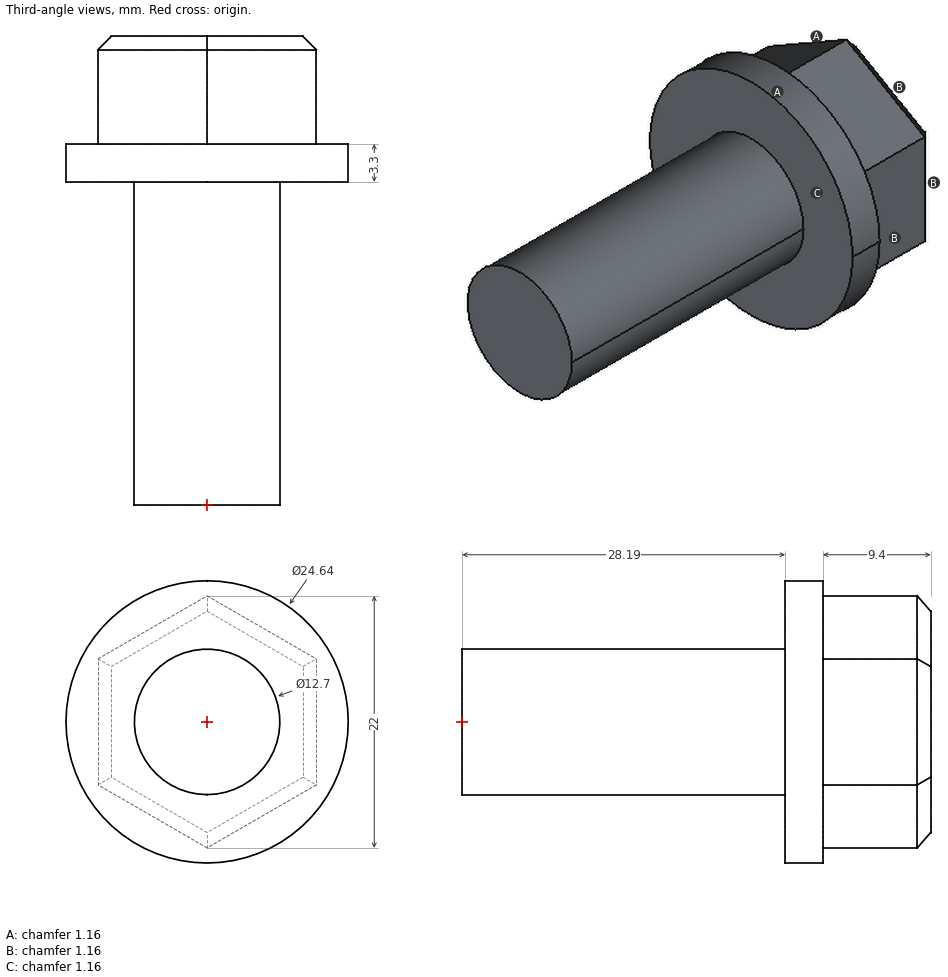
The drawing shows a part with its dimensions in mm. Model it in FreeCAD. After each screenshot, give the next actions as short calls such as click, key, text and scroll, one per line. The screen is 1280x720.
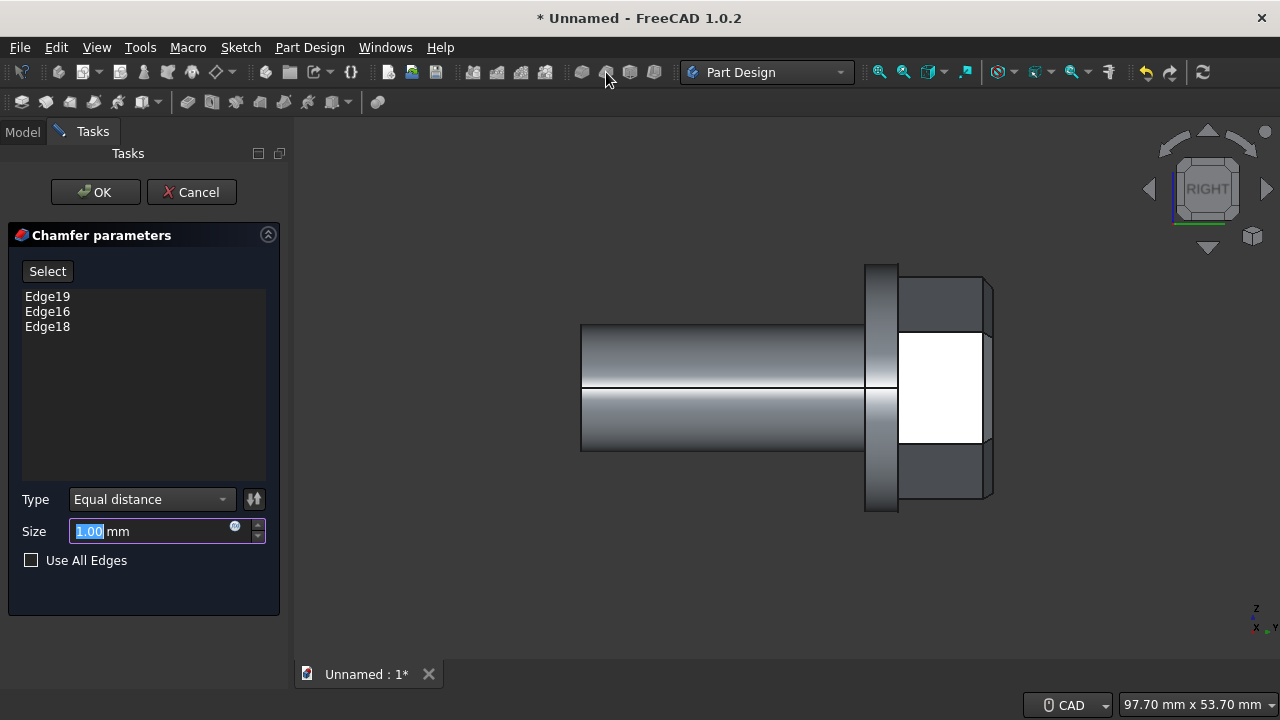
text(1.16)
key(Tab)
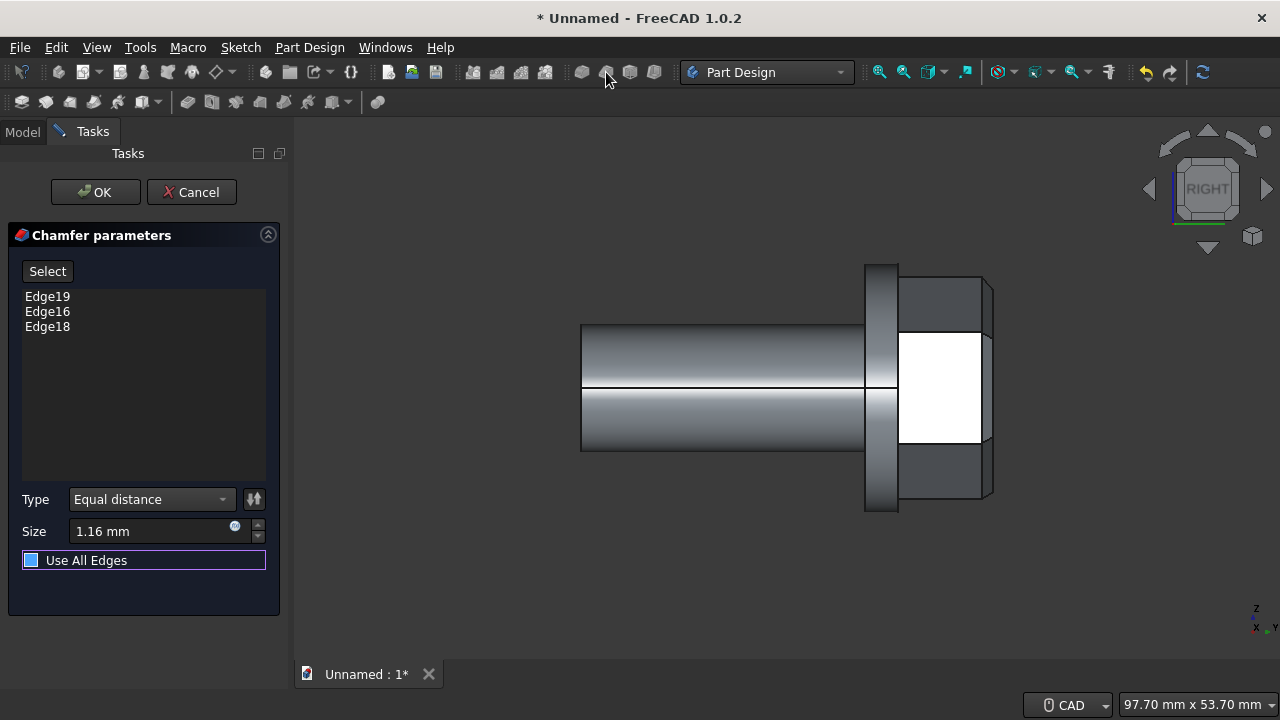
click(96, 192)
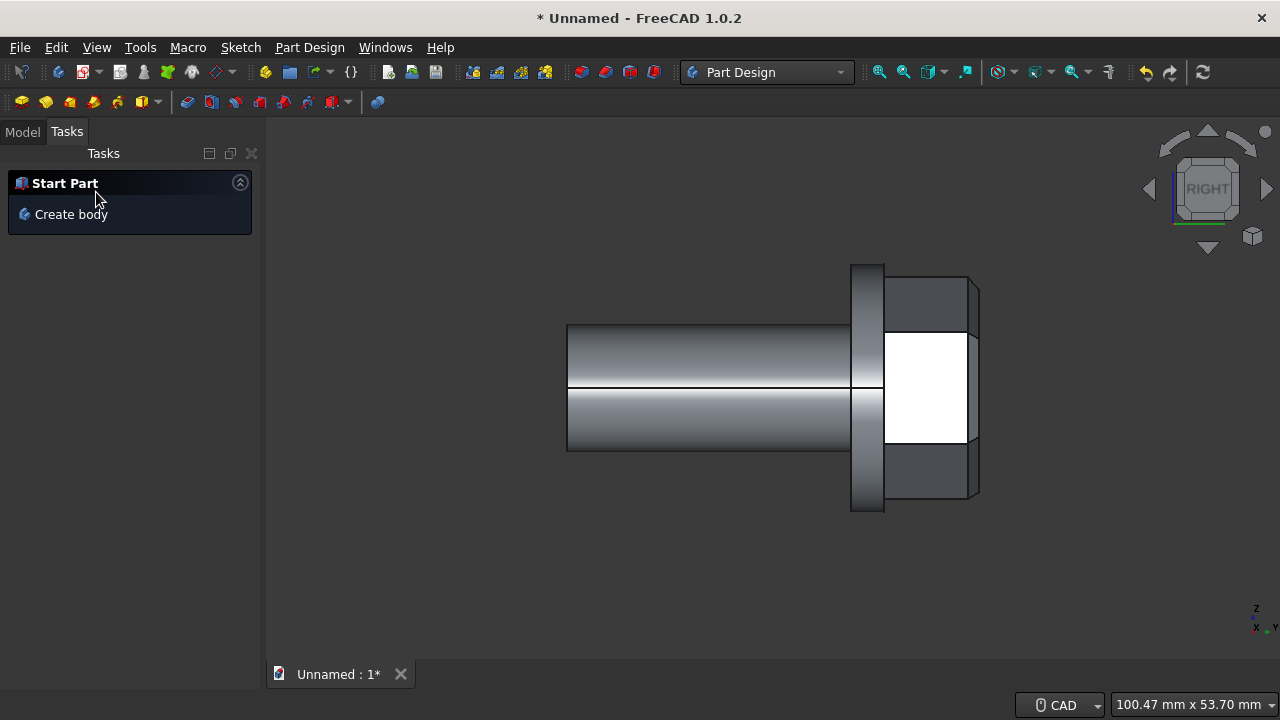
key(0)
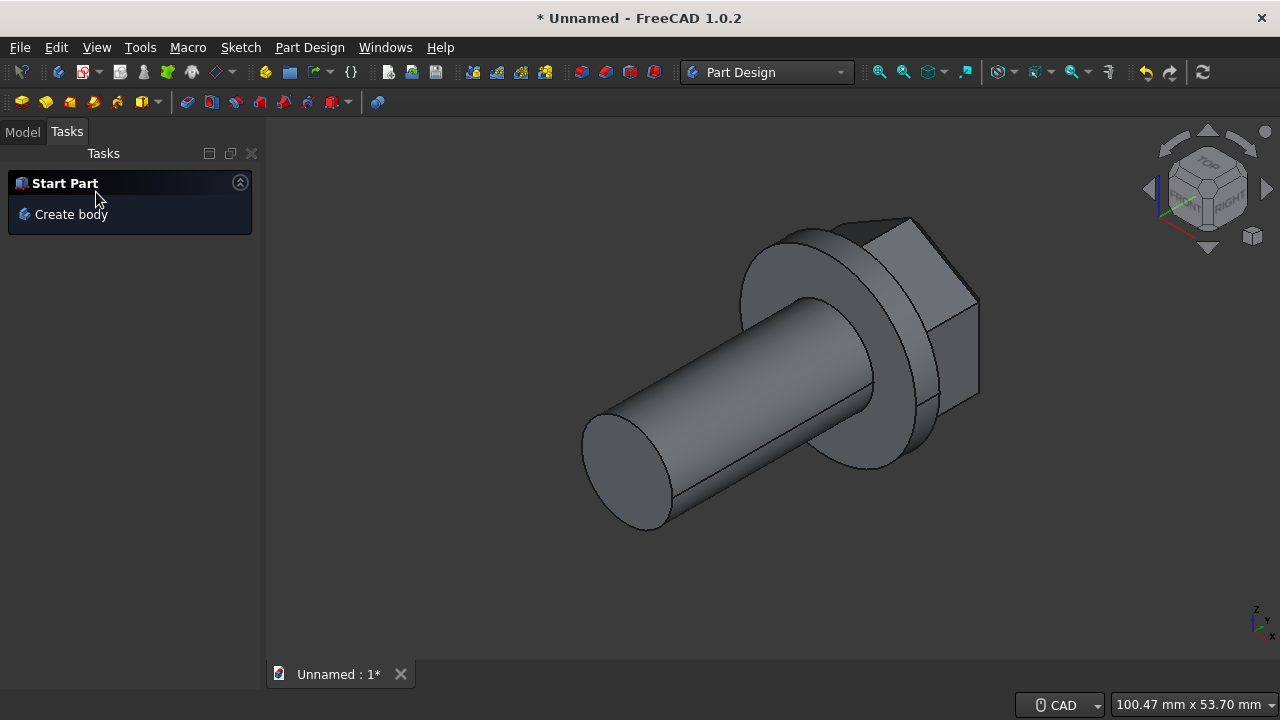
key(2)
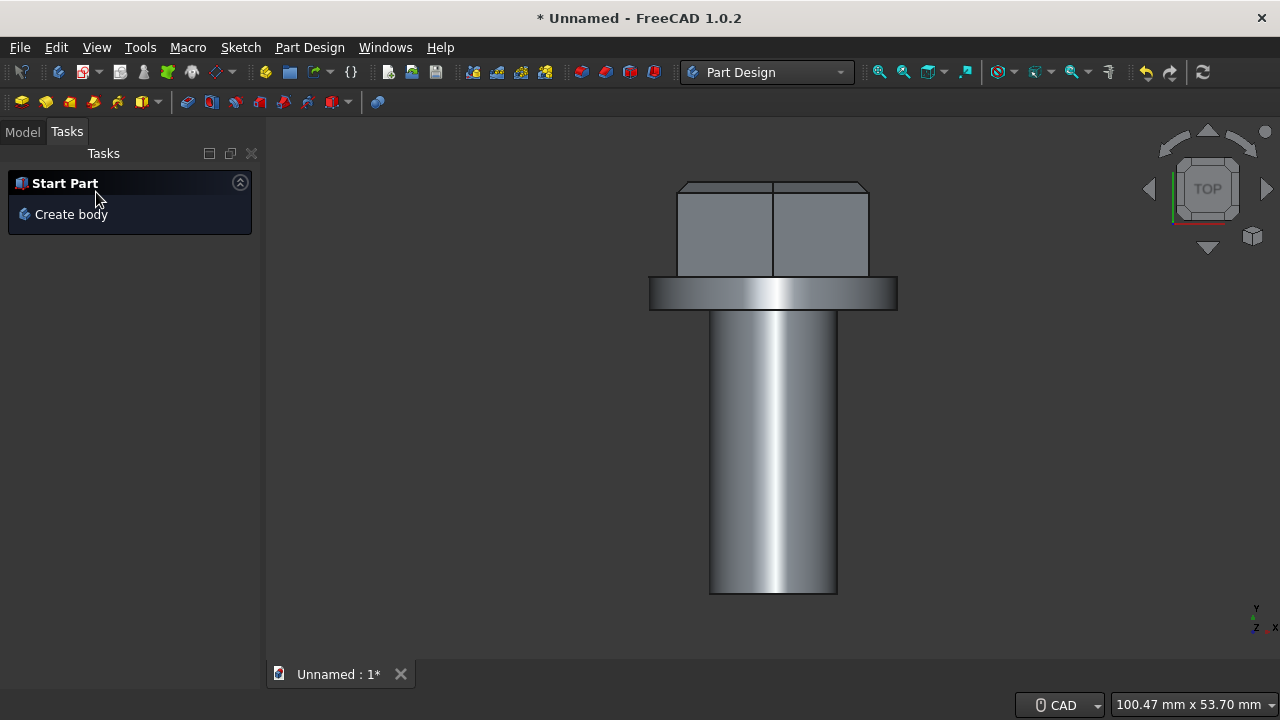
key(1)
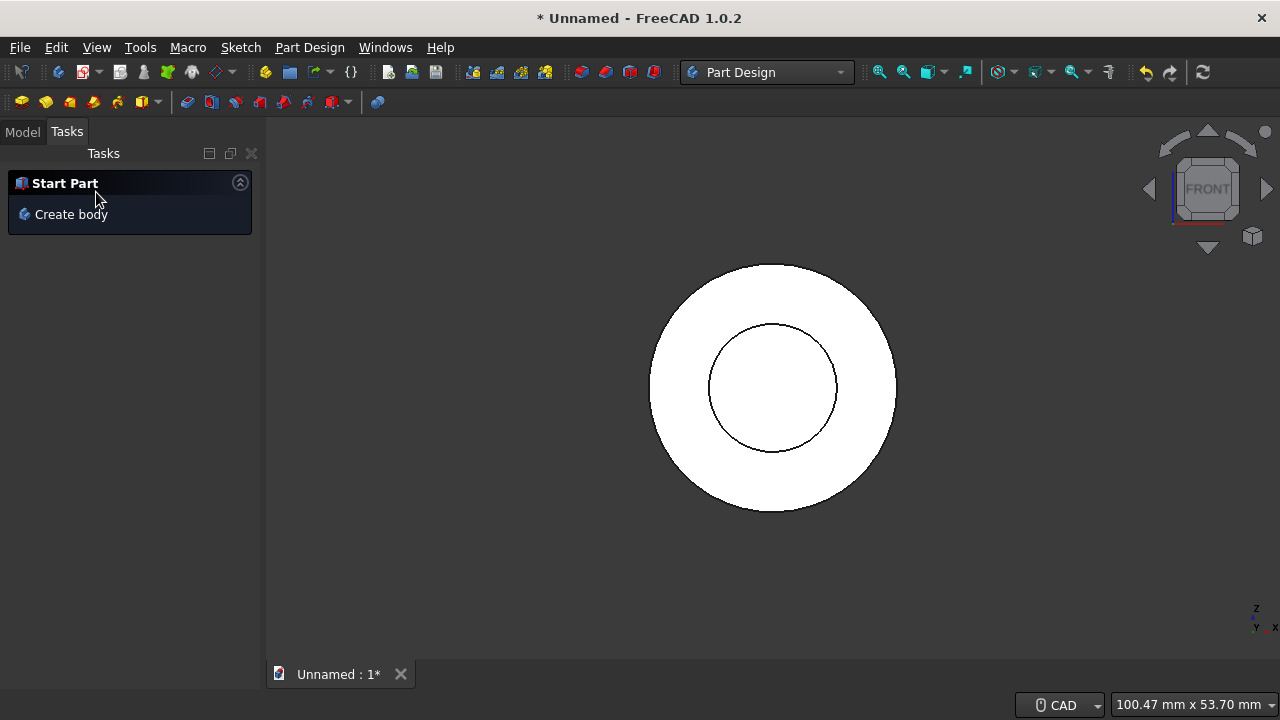
key(3)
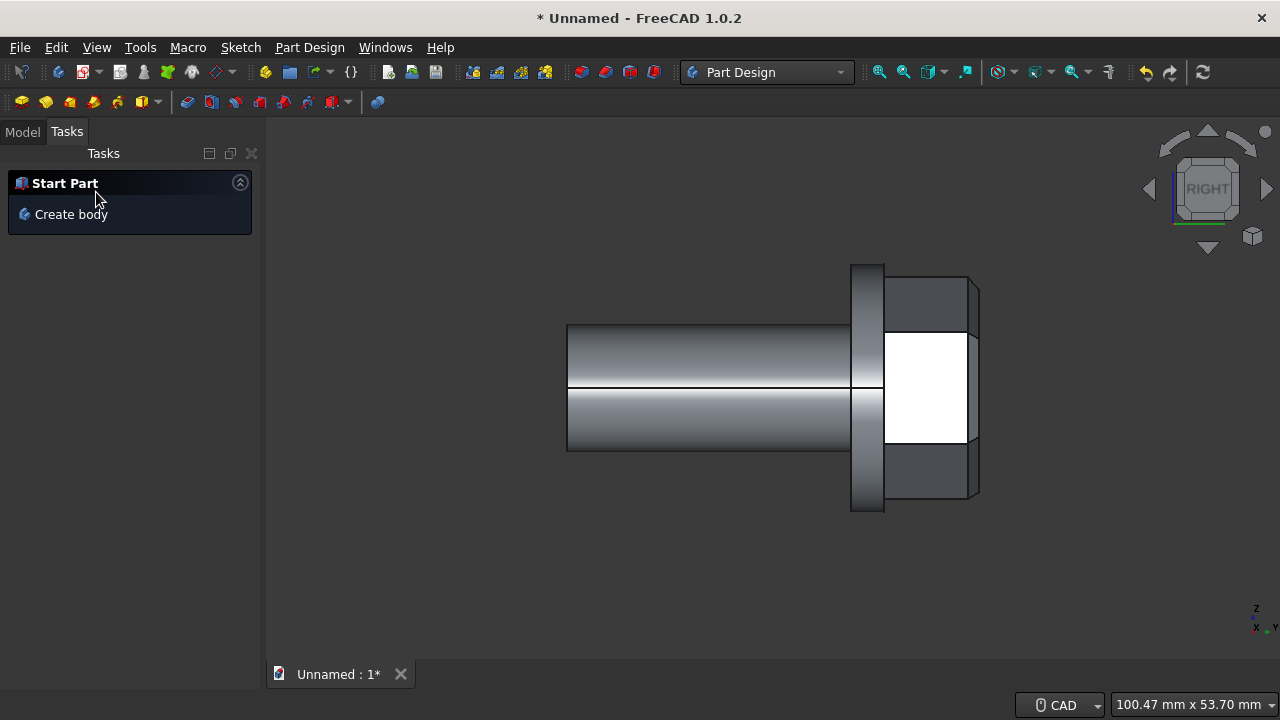
key(5)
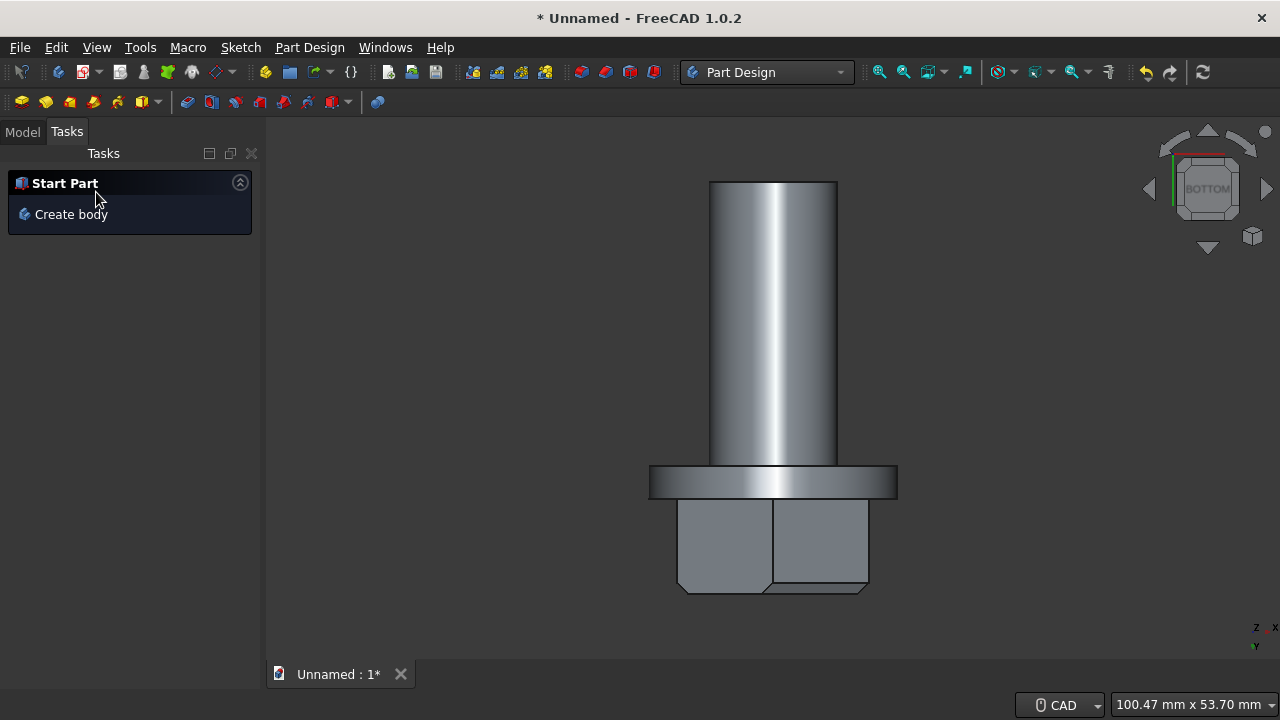
key(4)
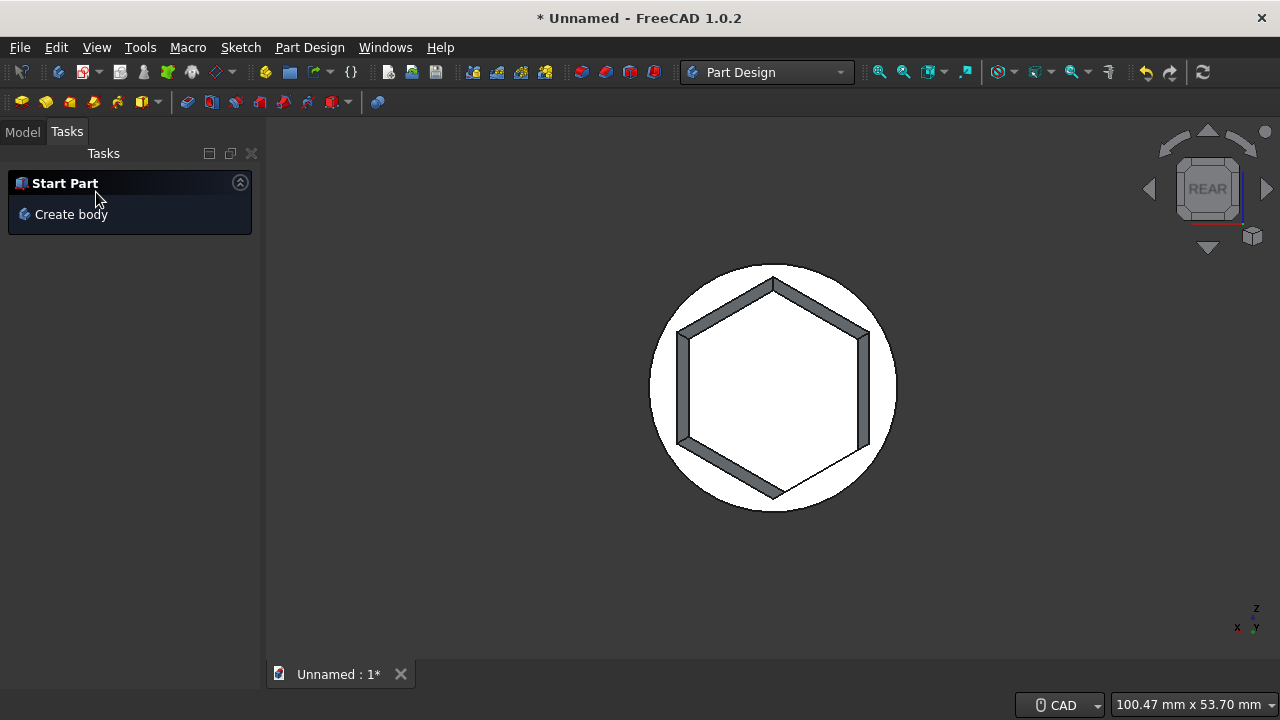
click(821, 470)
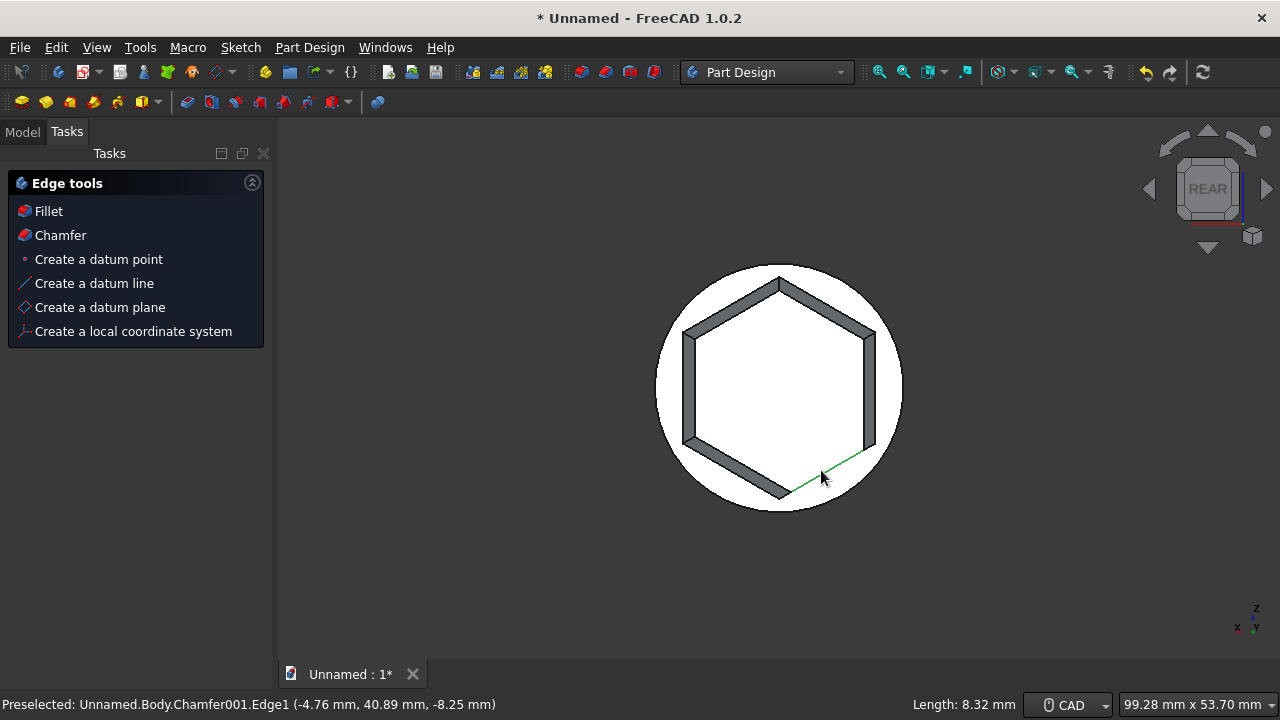
click(606, 72)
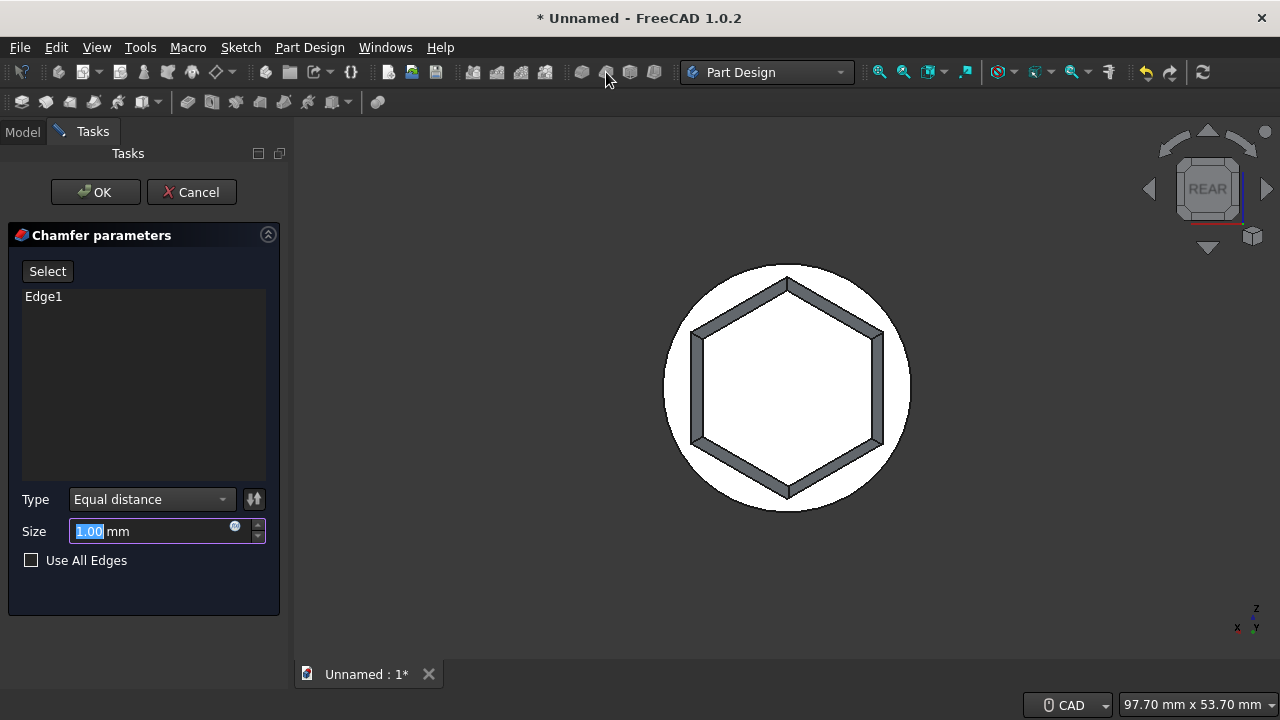
text(1.16)
key(Tab)